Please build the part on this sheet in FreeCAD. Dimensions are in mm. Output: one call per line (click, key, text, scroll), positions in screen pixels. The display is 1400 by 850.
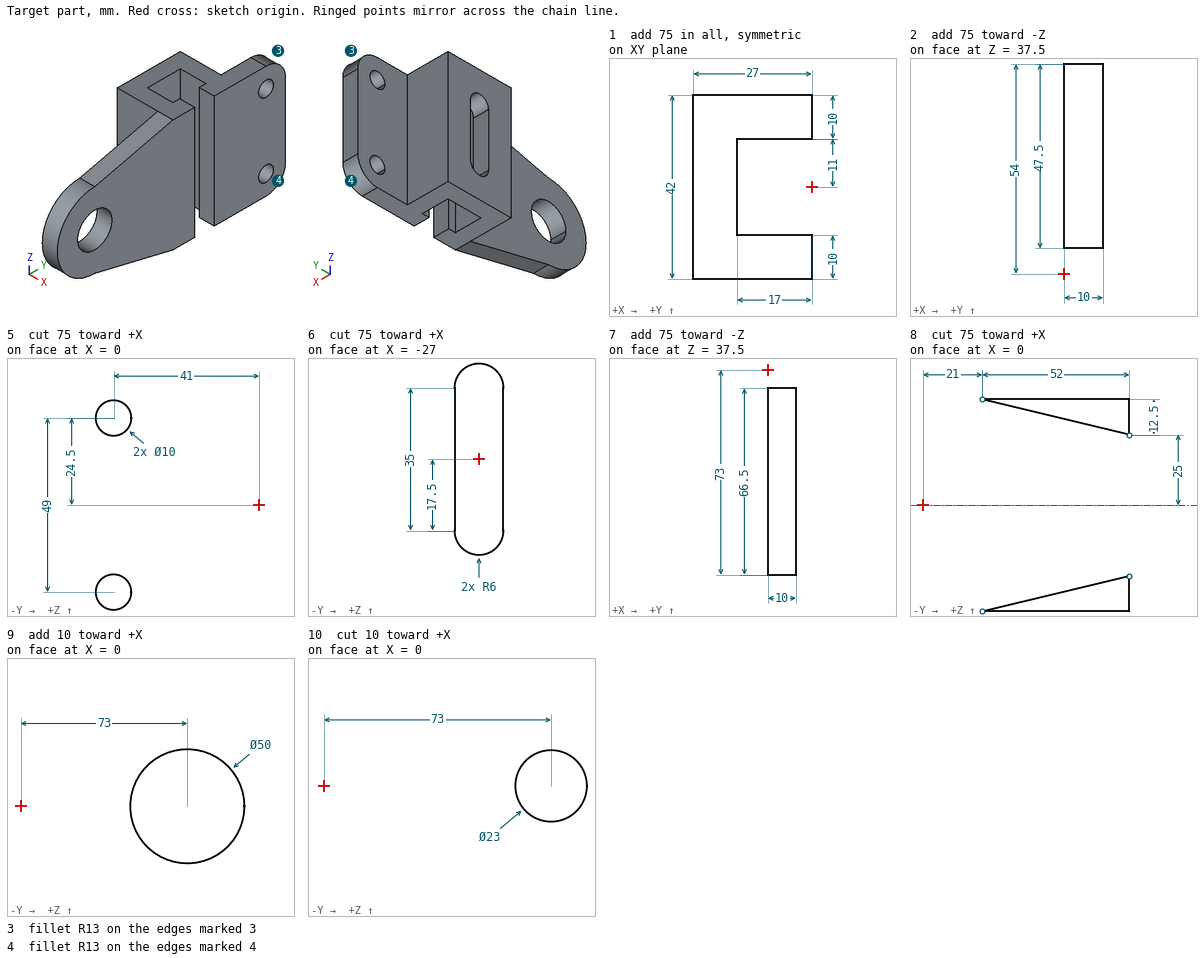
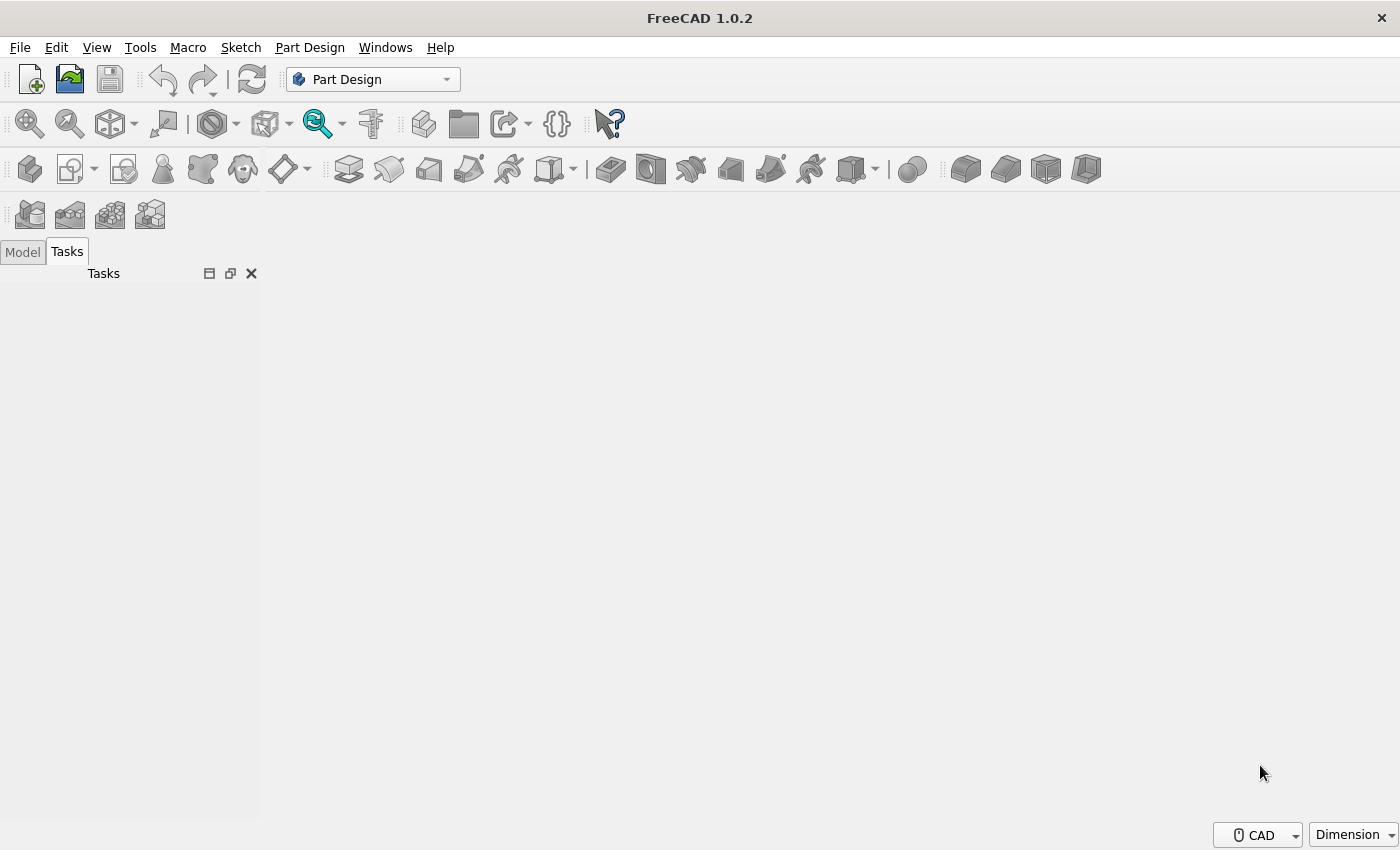
click(522, 80)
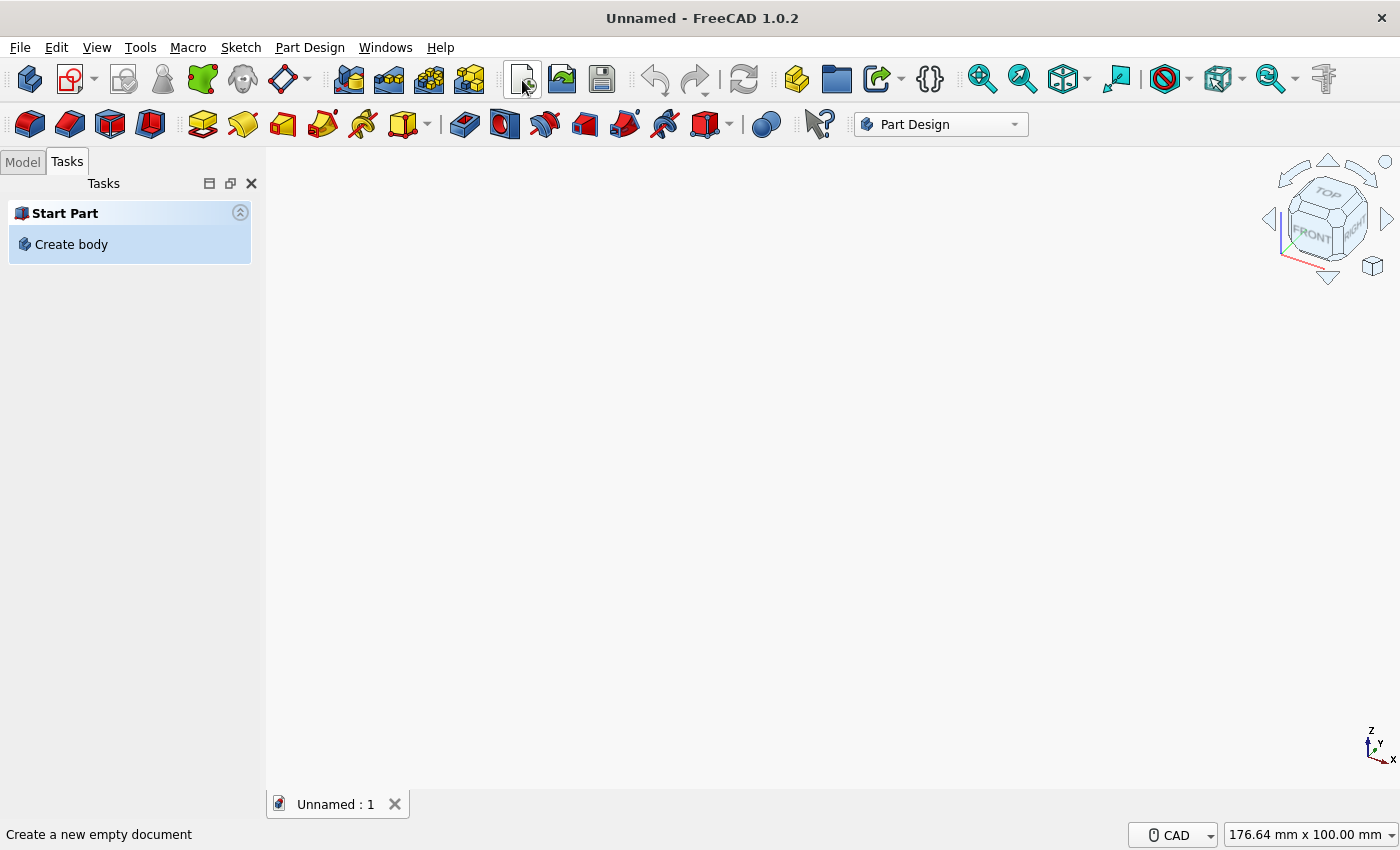
click(70, 80)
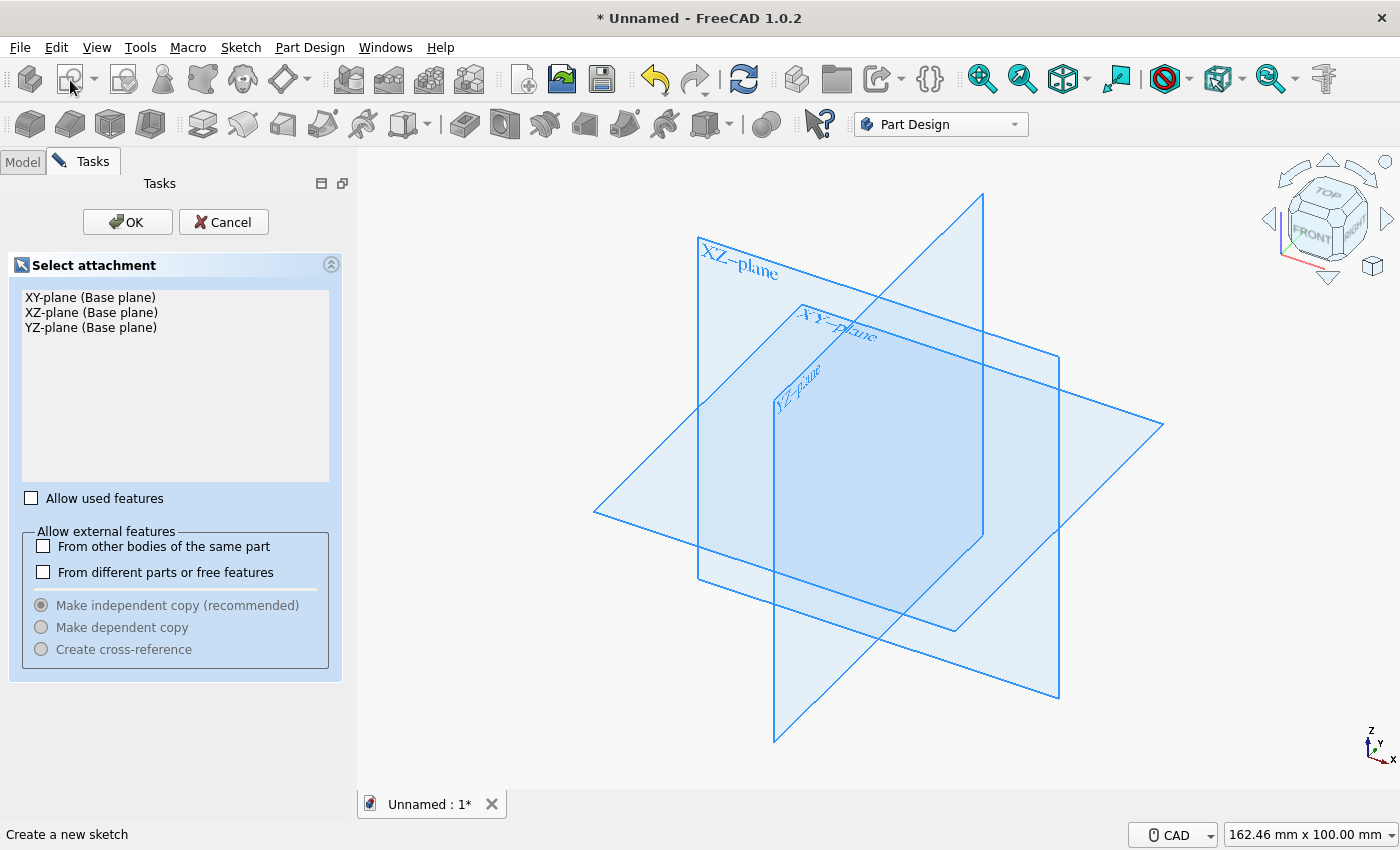
click(82, 298)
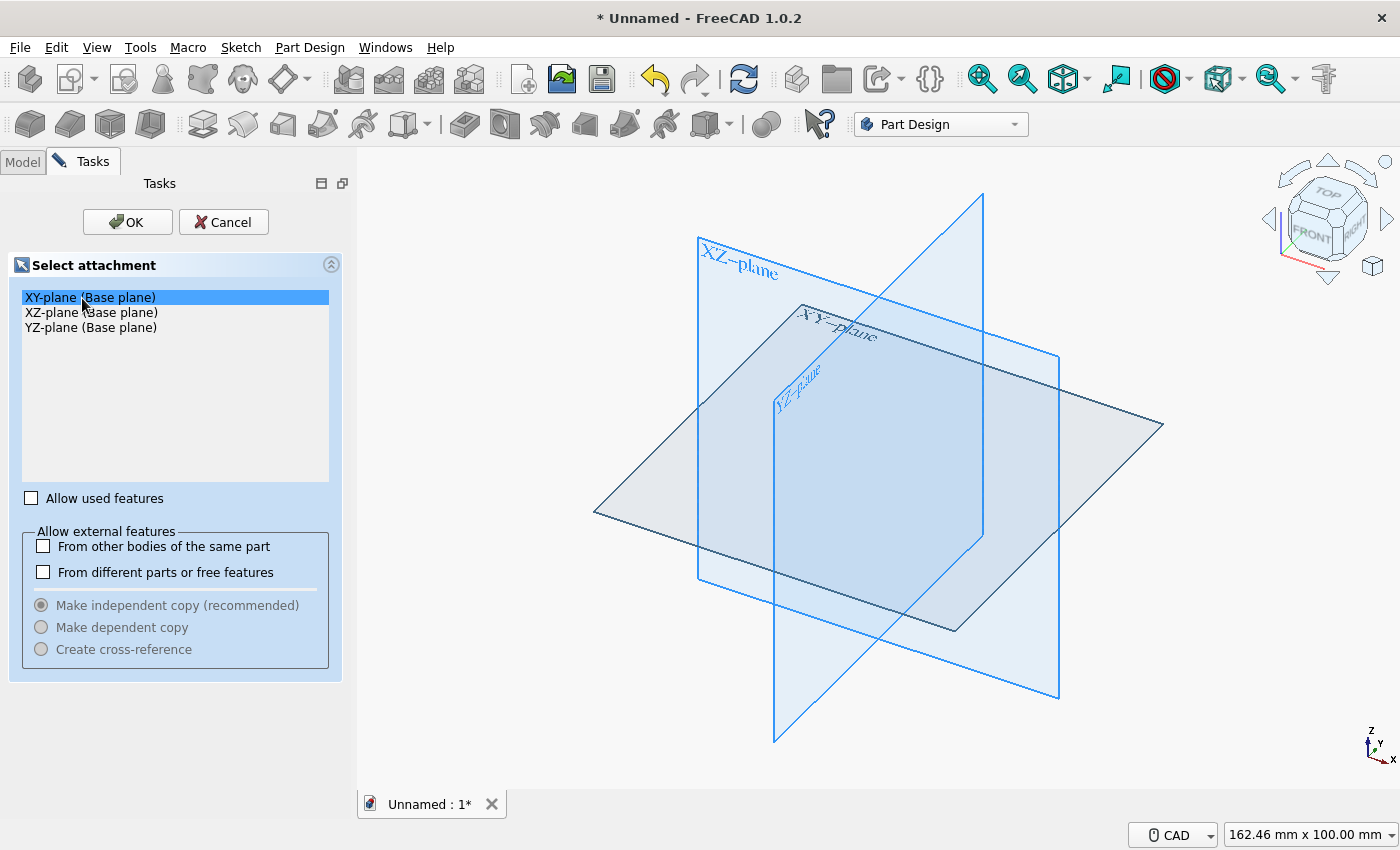
click(128, 222)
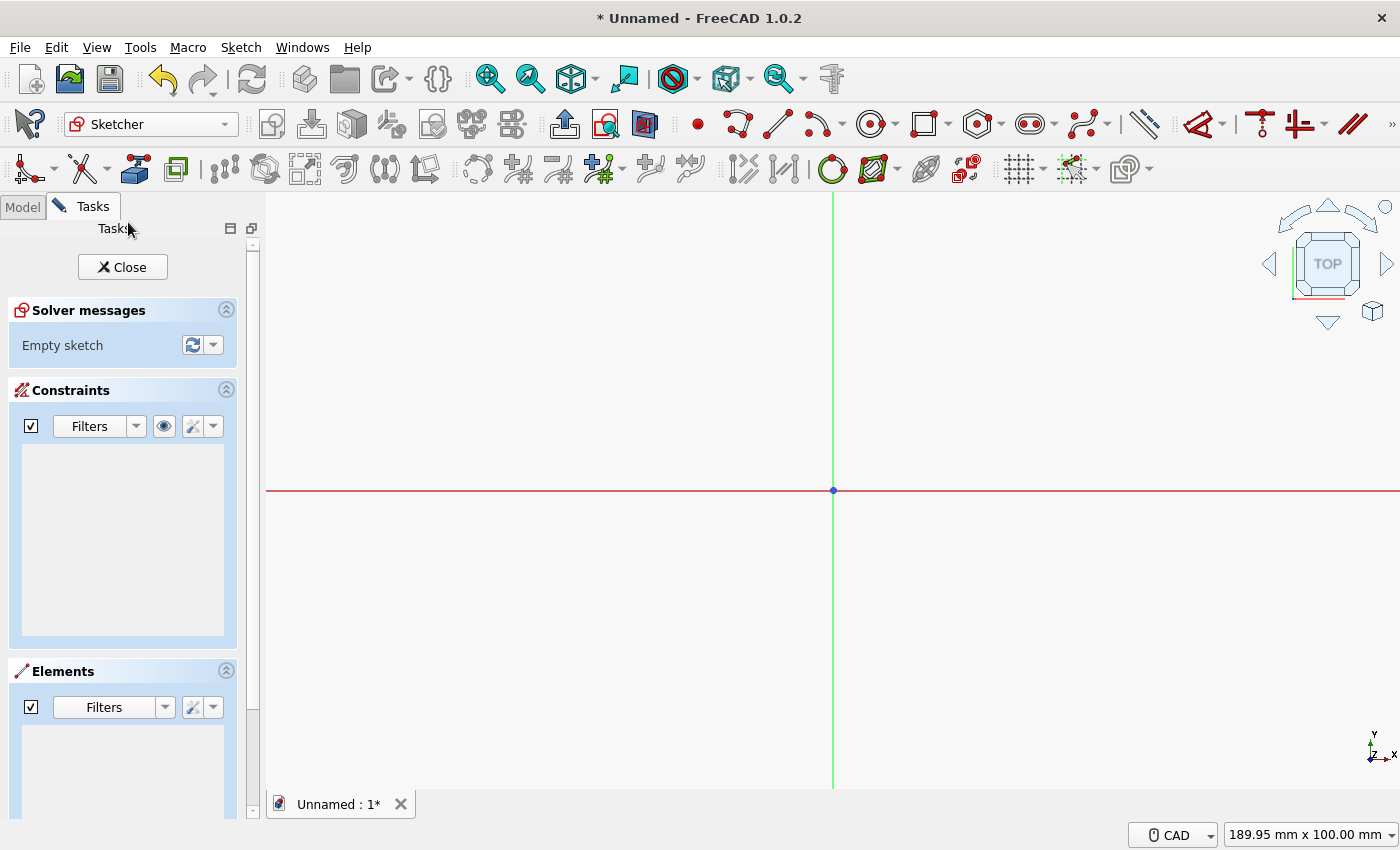
scroll(728, 490, up, 2)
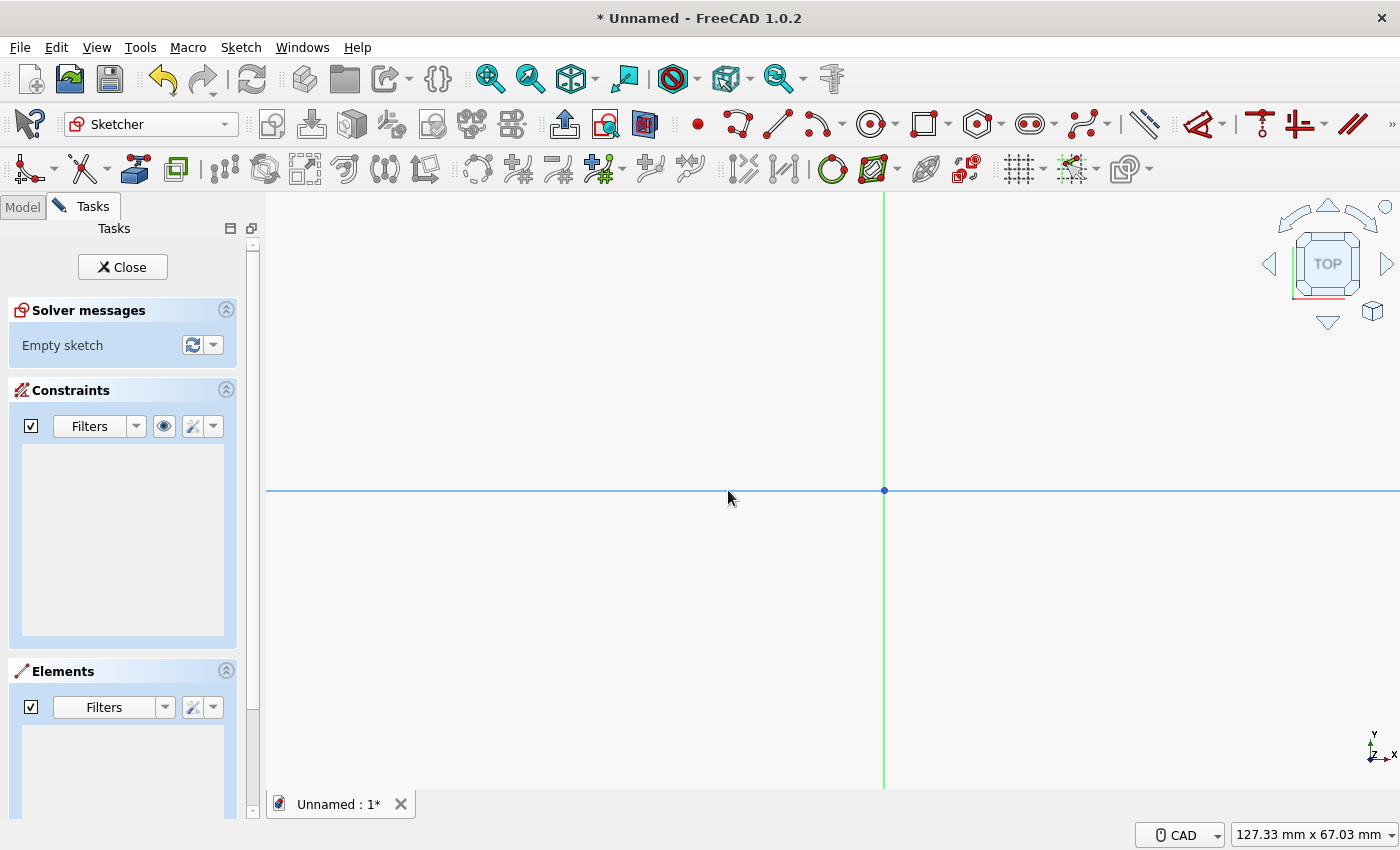
key(g)
key(m)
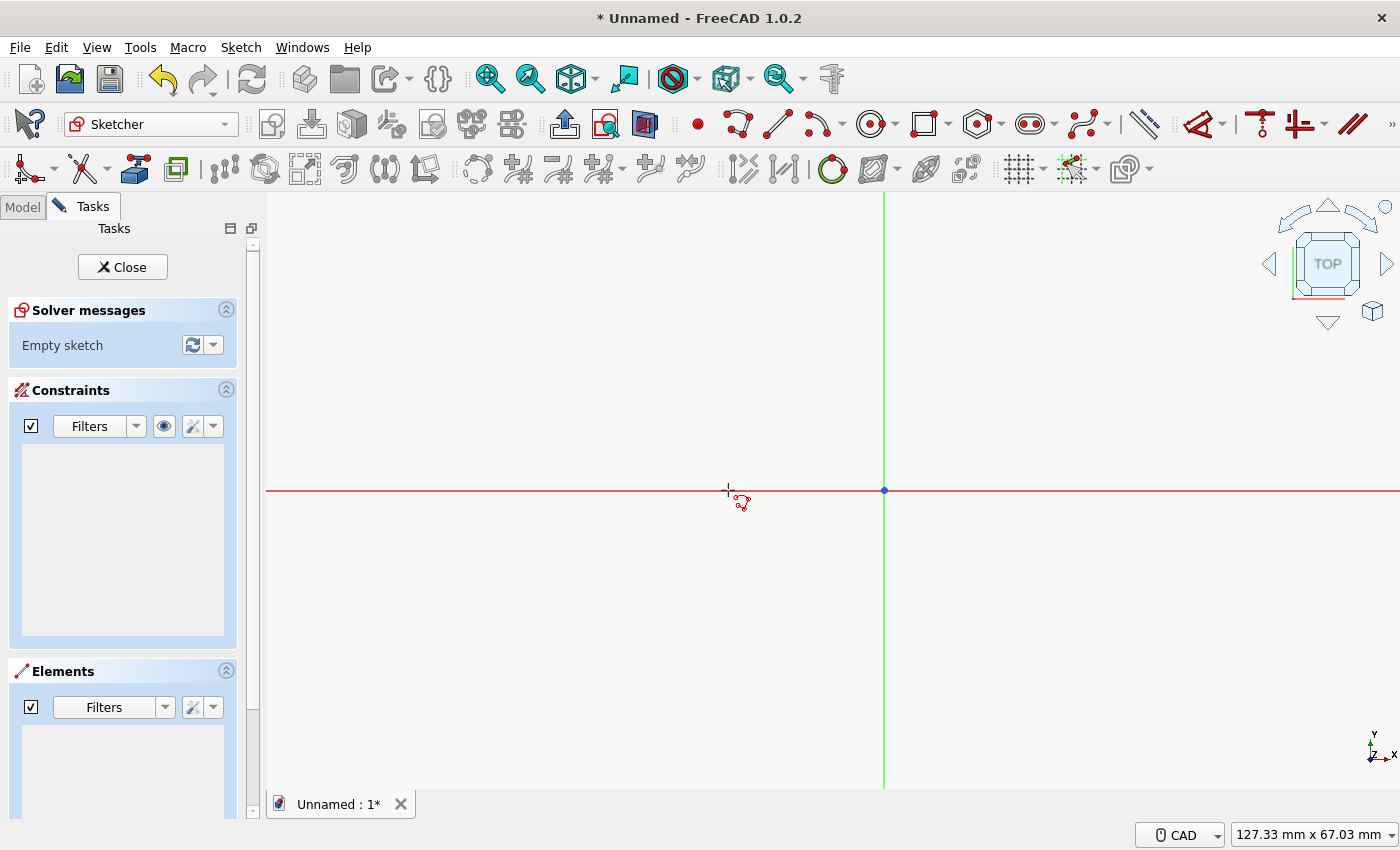
click(884, 393)
click(875, 303)
click(644, 303)
click(644, 678)
click(884, 678)
click(875, 588)
click(733, 588)
click(733, 393)
click(884, 394)
key(Escape)
key(Escape)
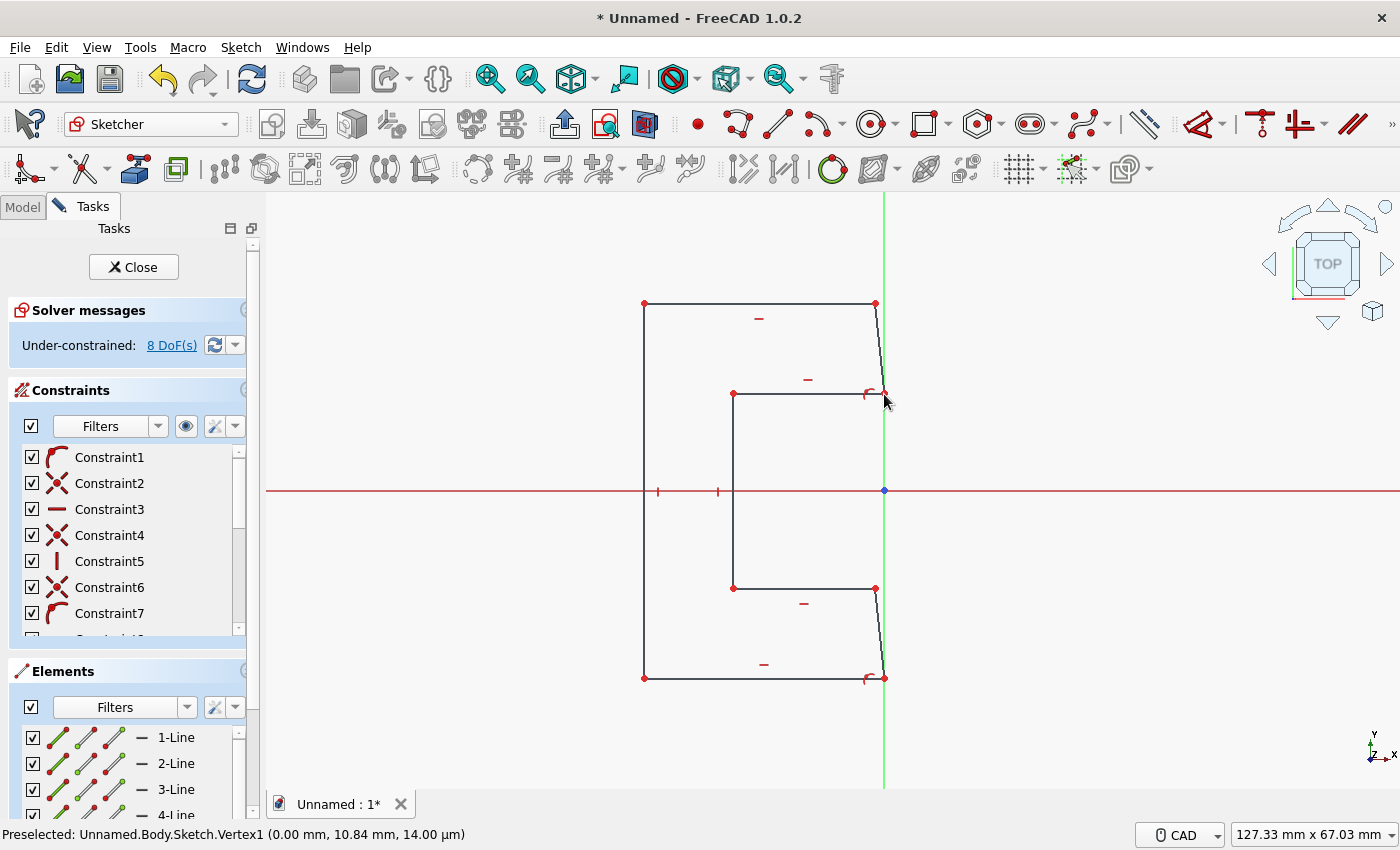
click(882, 367)